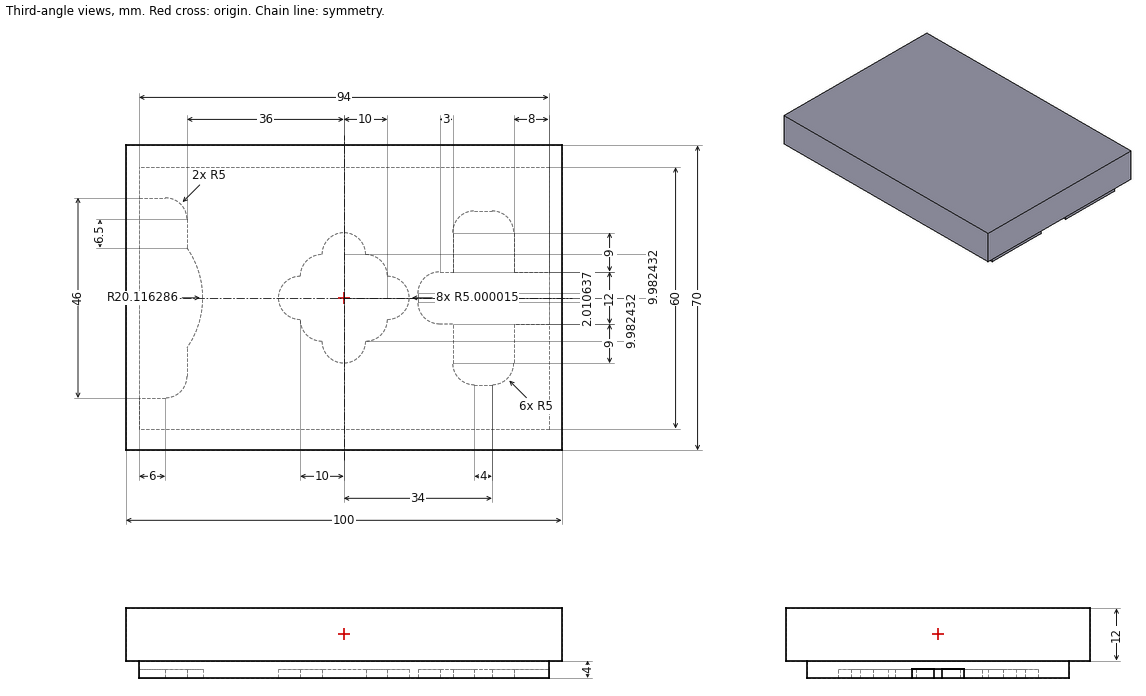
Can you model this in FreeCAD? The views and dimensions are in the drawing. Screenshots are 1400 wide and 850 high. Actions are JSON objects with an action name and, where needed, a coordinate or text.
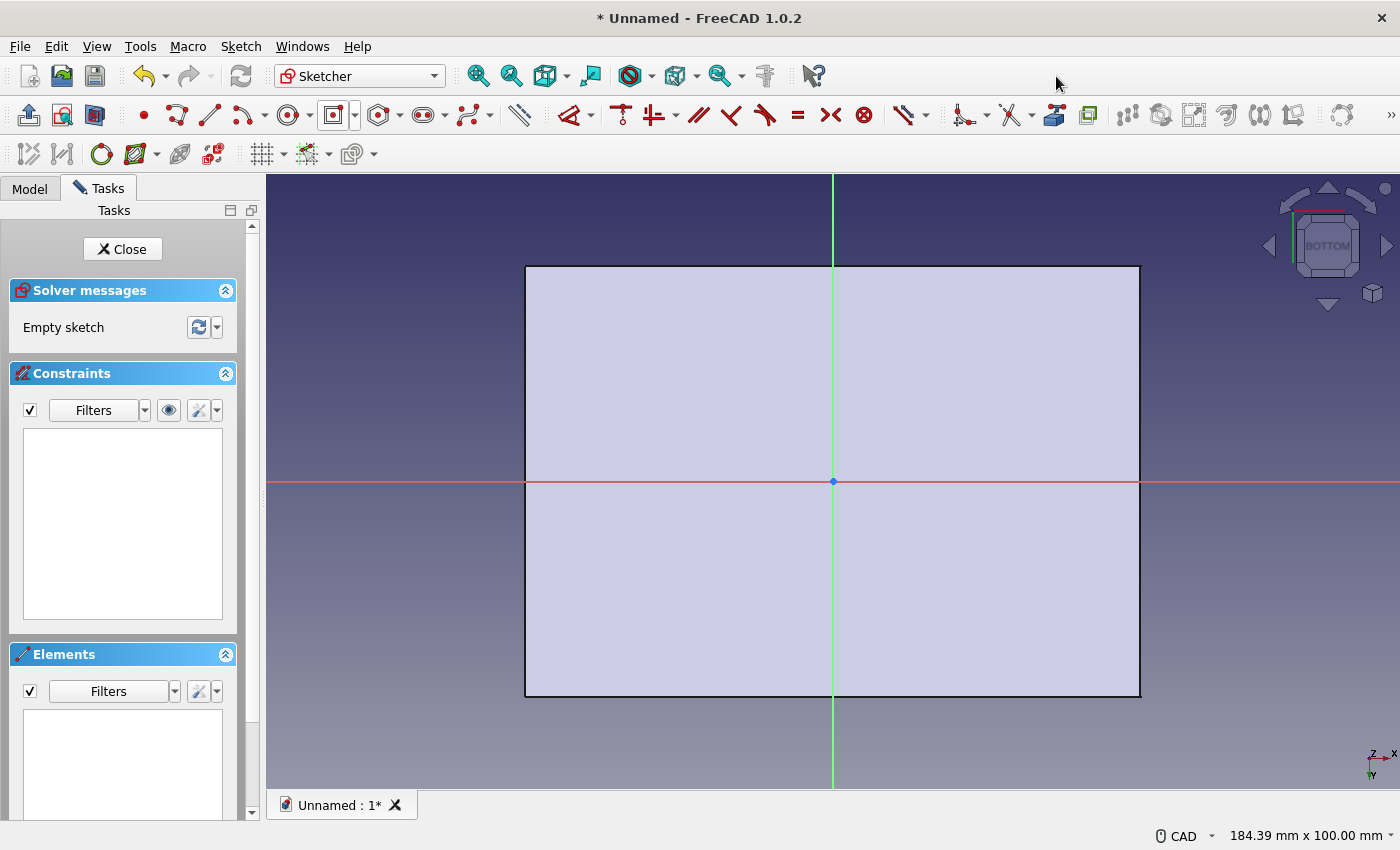
{"action": "left_click", "coordinate": [332, 116]}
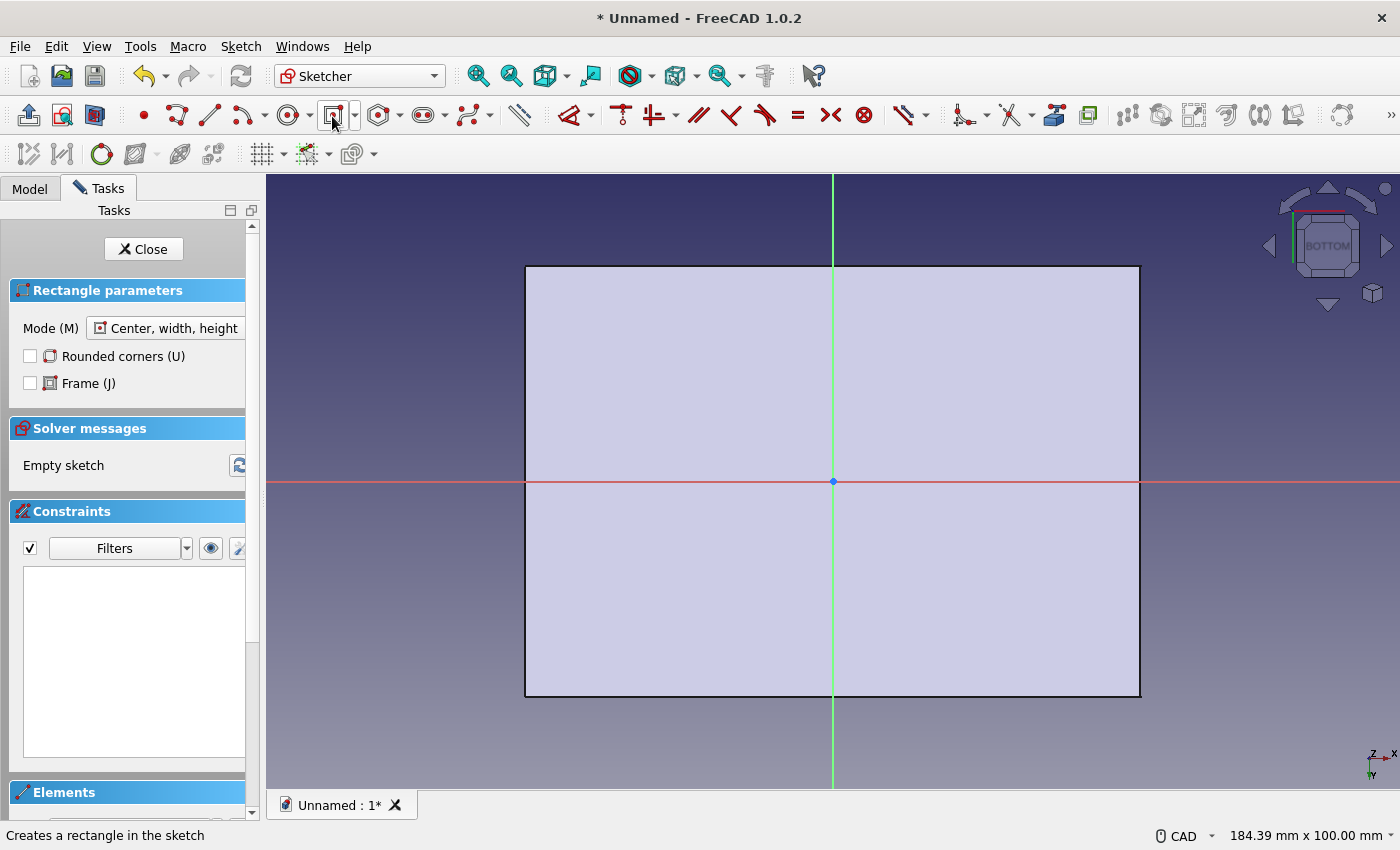
{"action": "left_click", "coordinate": [833, 482]}
{"action": "mouse_move", "coordinate": [1122, 297]}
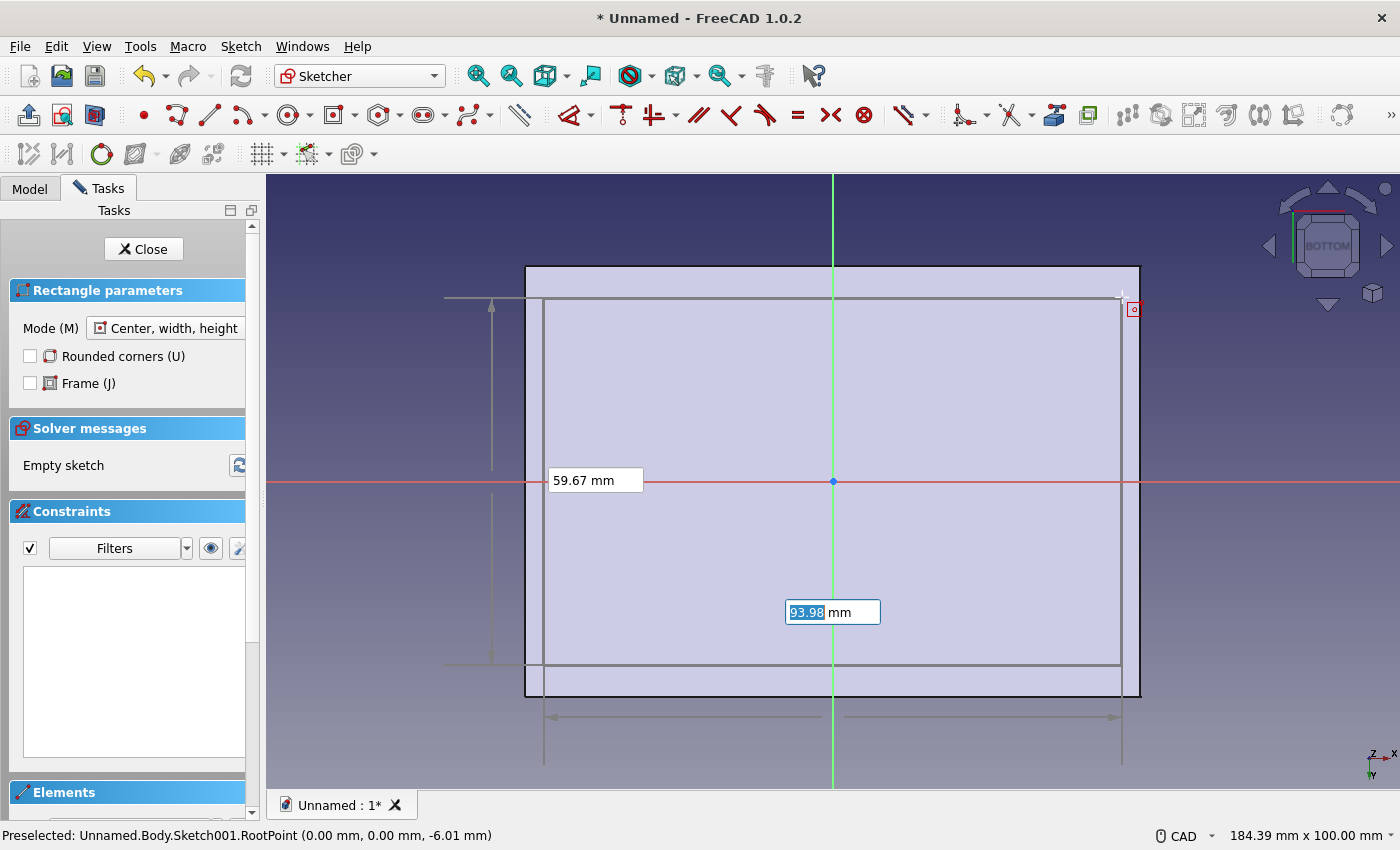
{"action": "type", "text": "94"}
{"action": "key", "text": "Tab"}
{"action": "type", "text": "60"}
{"action": "key", "text": "Return"}
{"action": "key", "text": "Escape"}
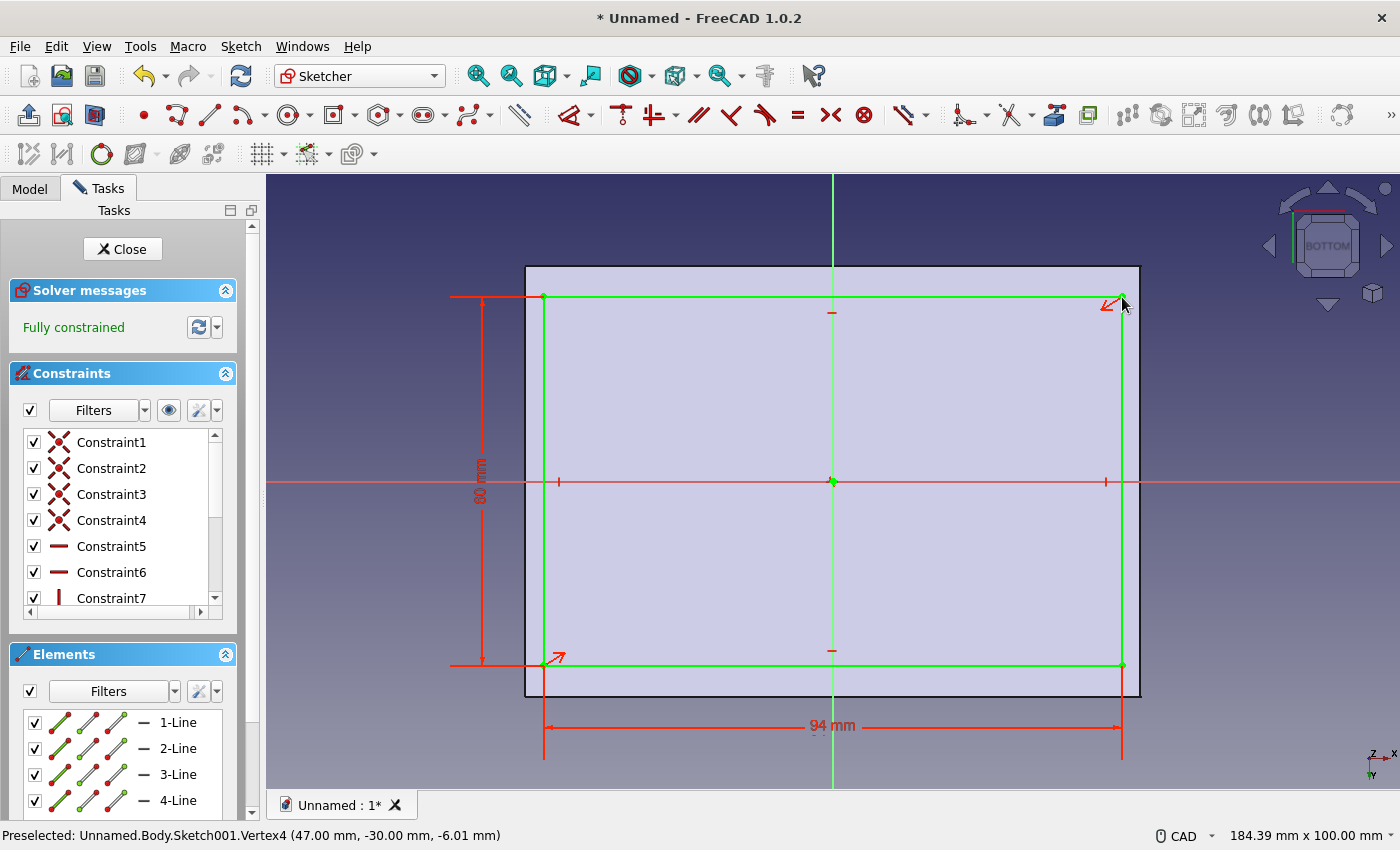
{"action": "left_click", "coordinate": [123, 249]}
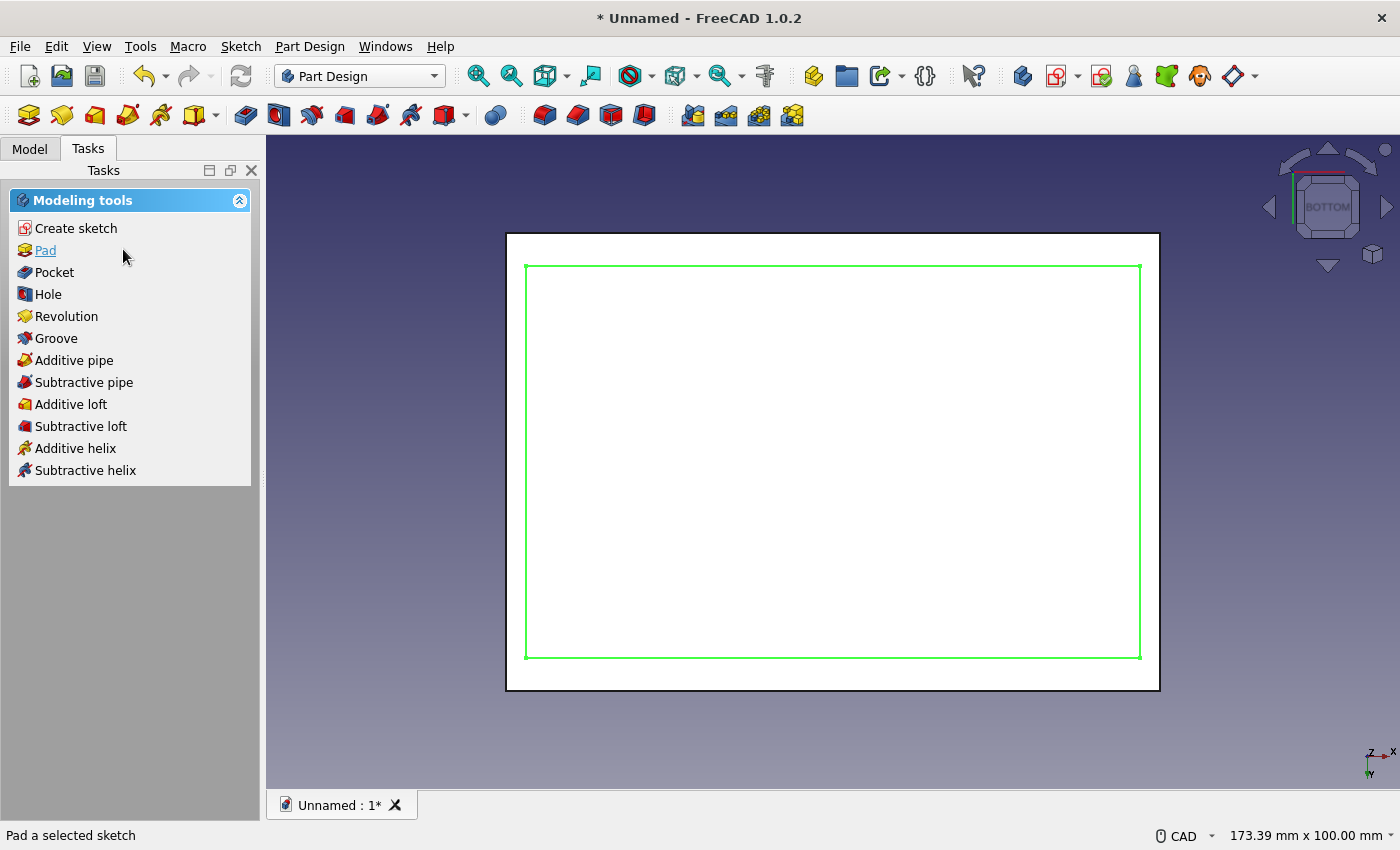
{"action": "left_click", "coordinate": [29, 116]}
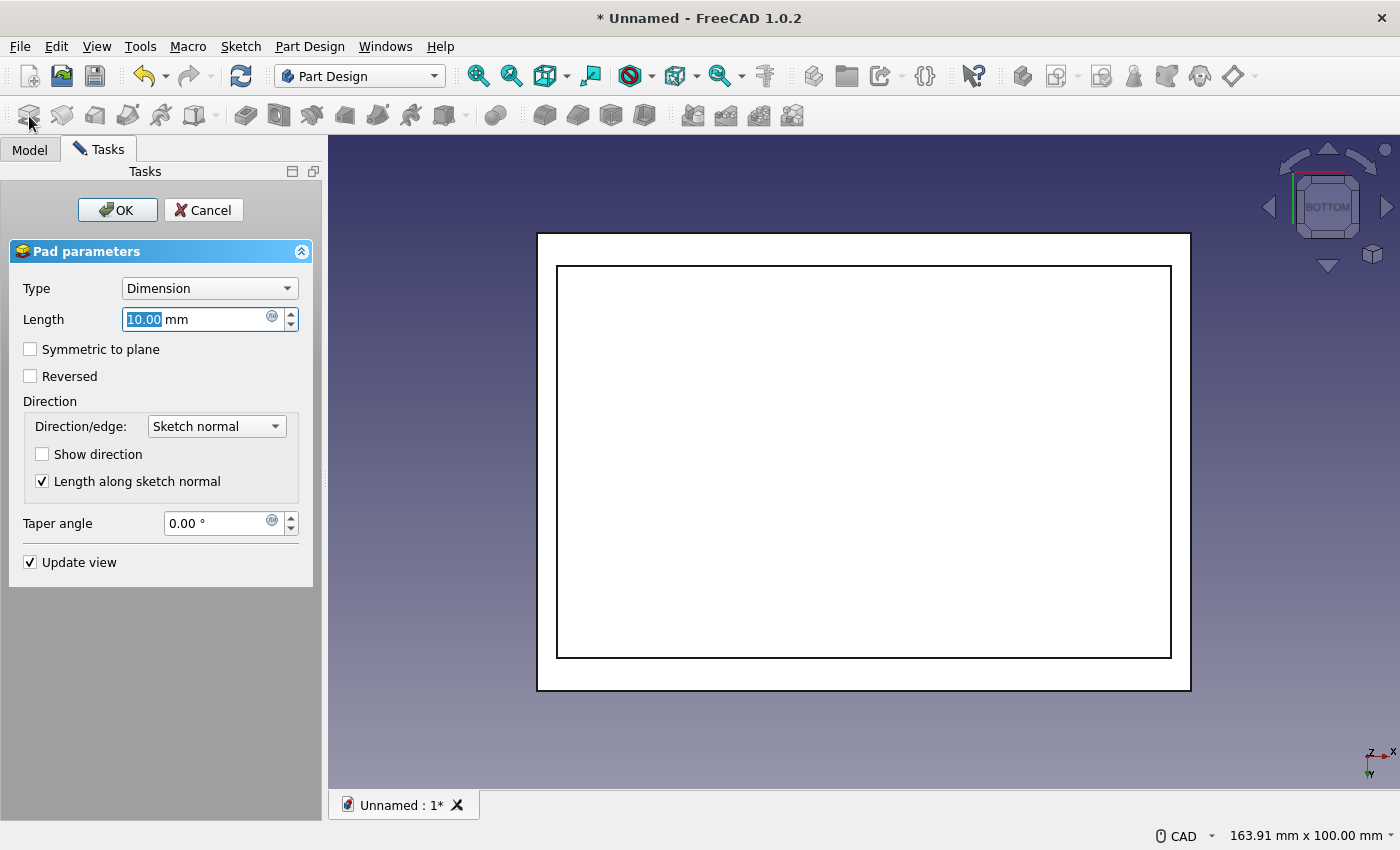
{"action": "type", "text": "4"}
{"action": "key", "text": "Tab"}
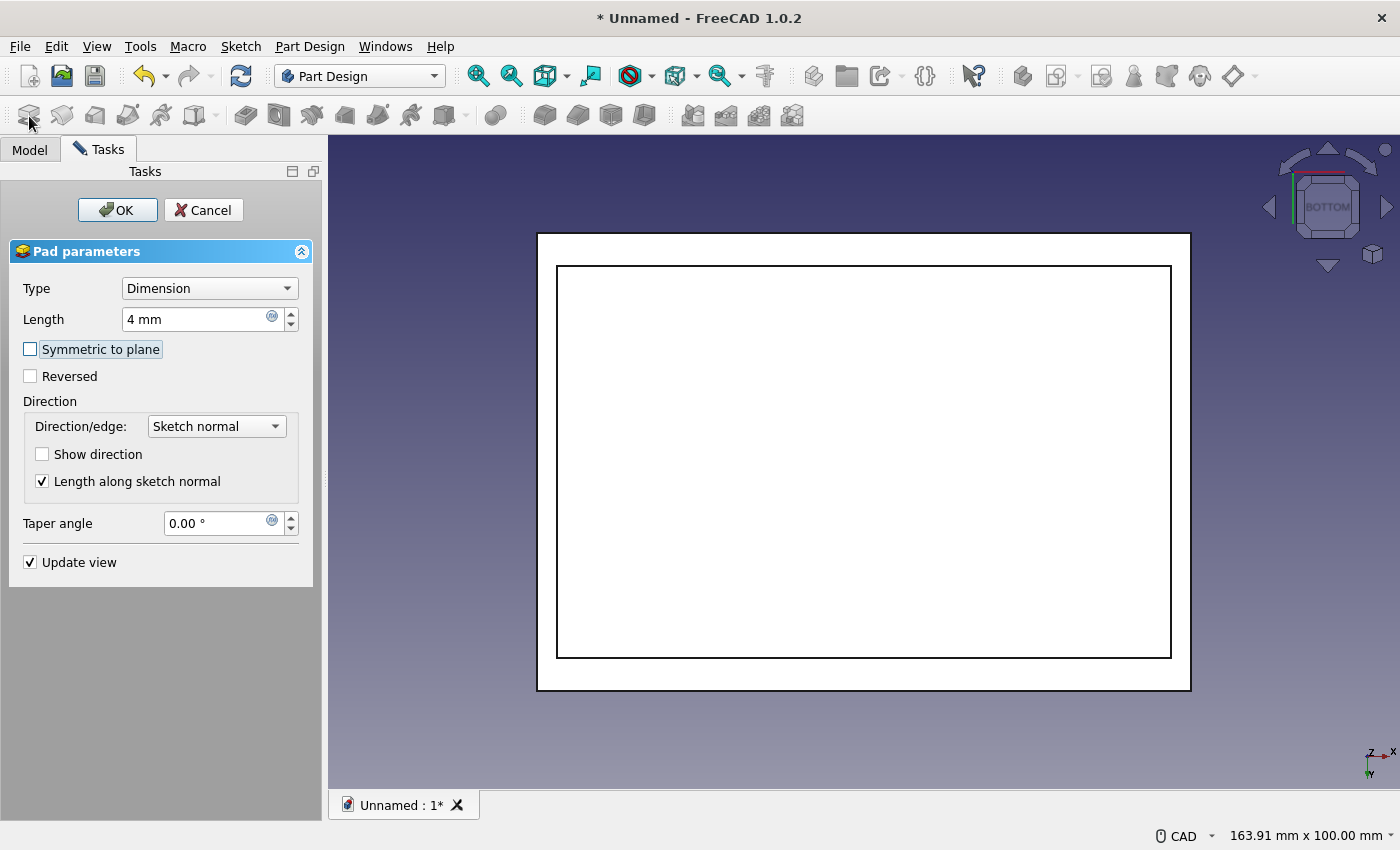
{"action": "left_click", "coordinate": [118, 210]}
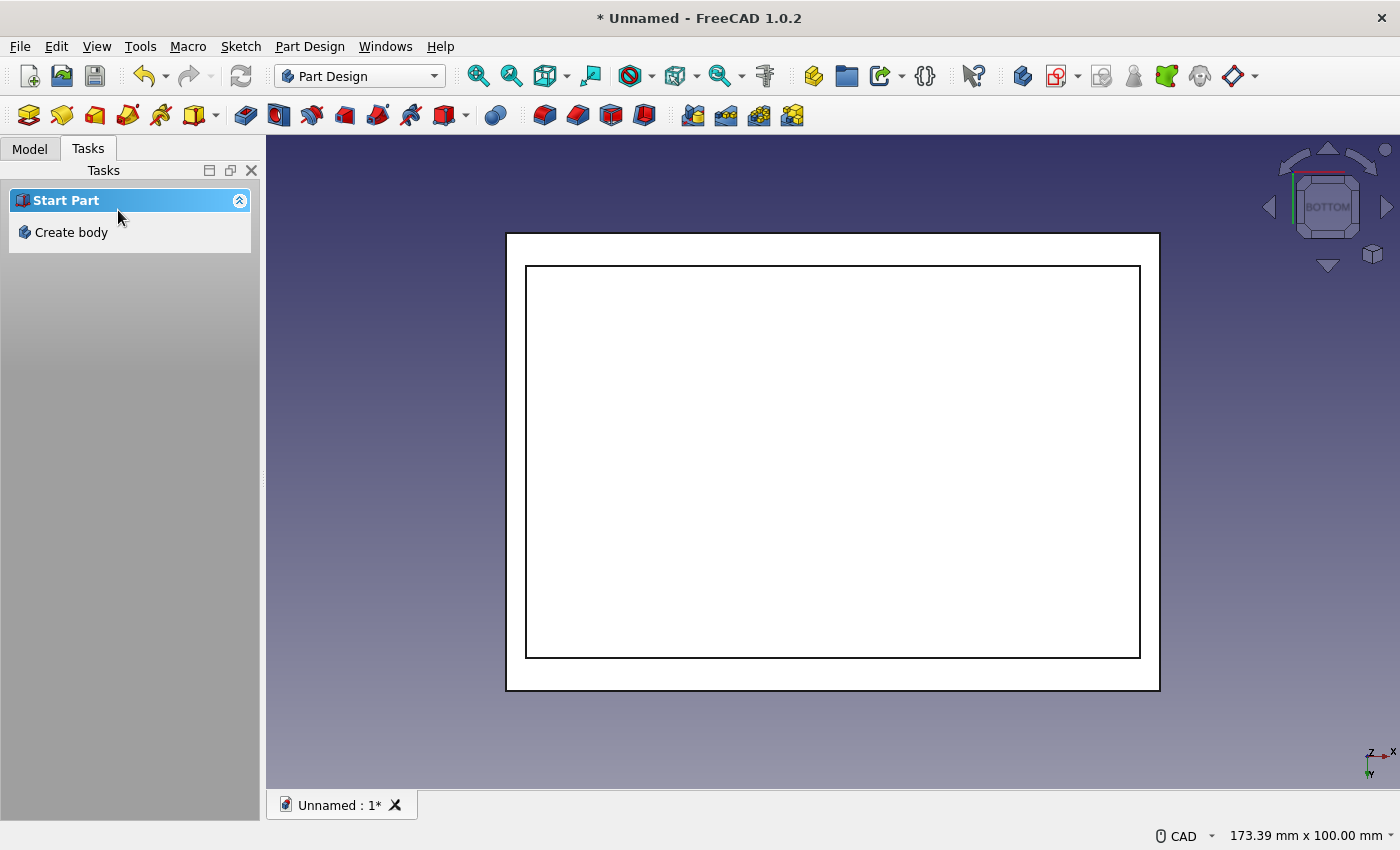
{"action": "left_click", "coordinate": [921, 461]}